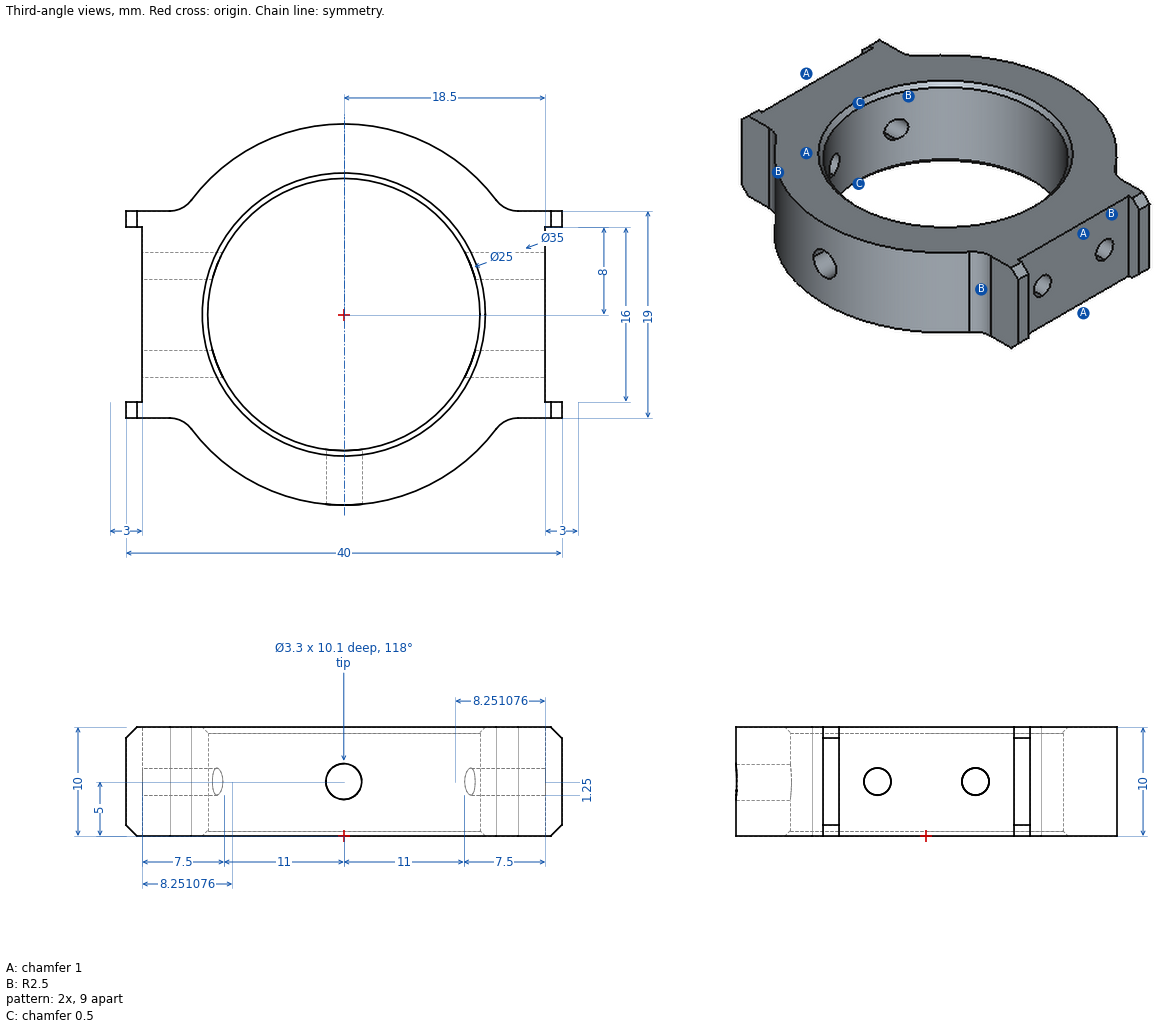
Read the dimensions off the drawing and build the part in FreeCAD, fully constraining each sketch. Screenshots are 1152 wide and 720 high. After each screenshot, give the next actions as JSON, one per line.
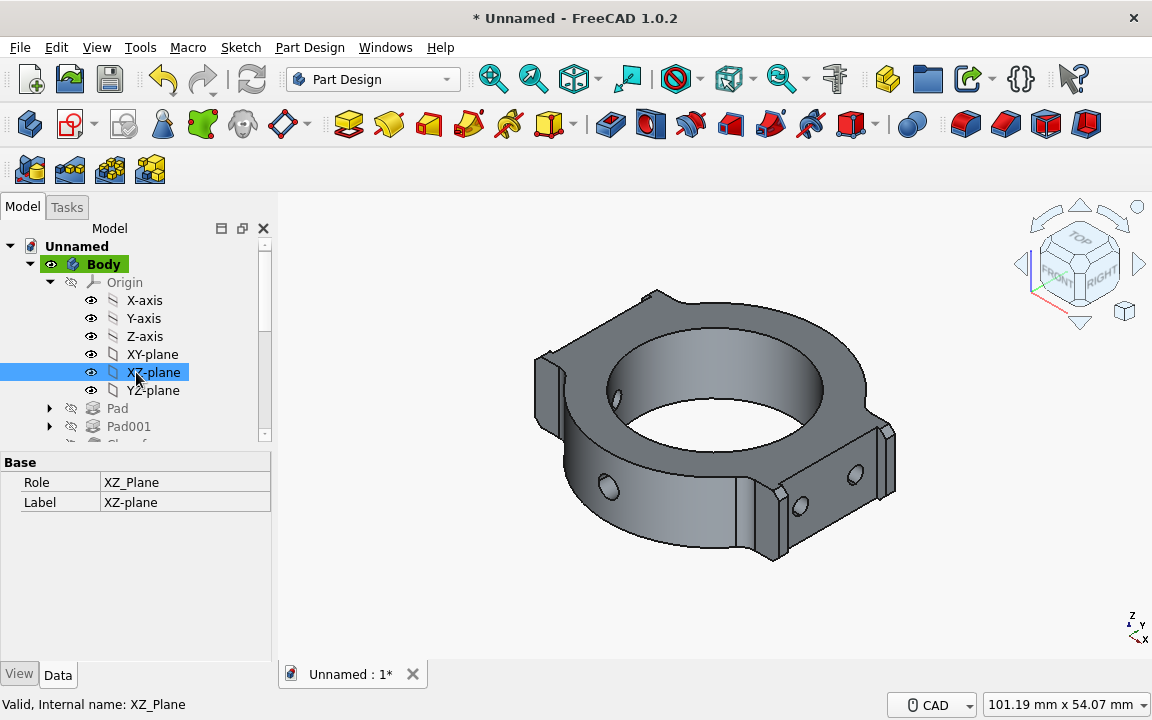
{"action": "left_click", "coordinate": [284, 124]}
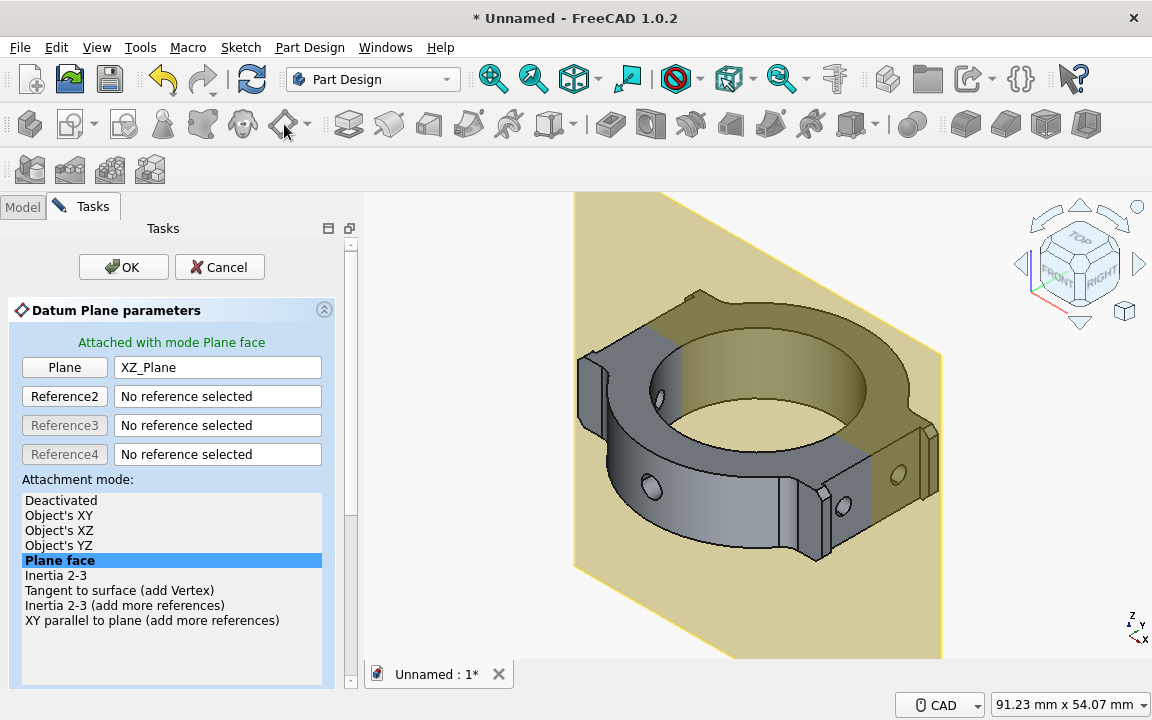
{"action": "scroll", "coordinate": [351, 463], "scroll_direction": "down", "scroll_amount": 3}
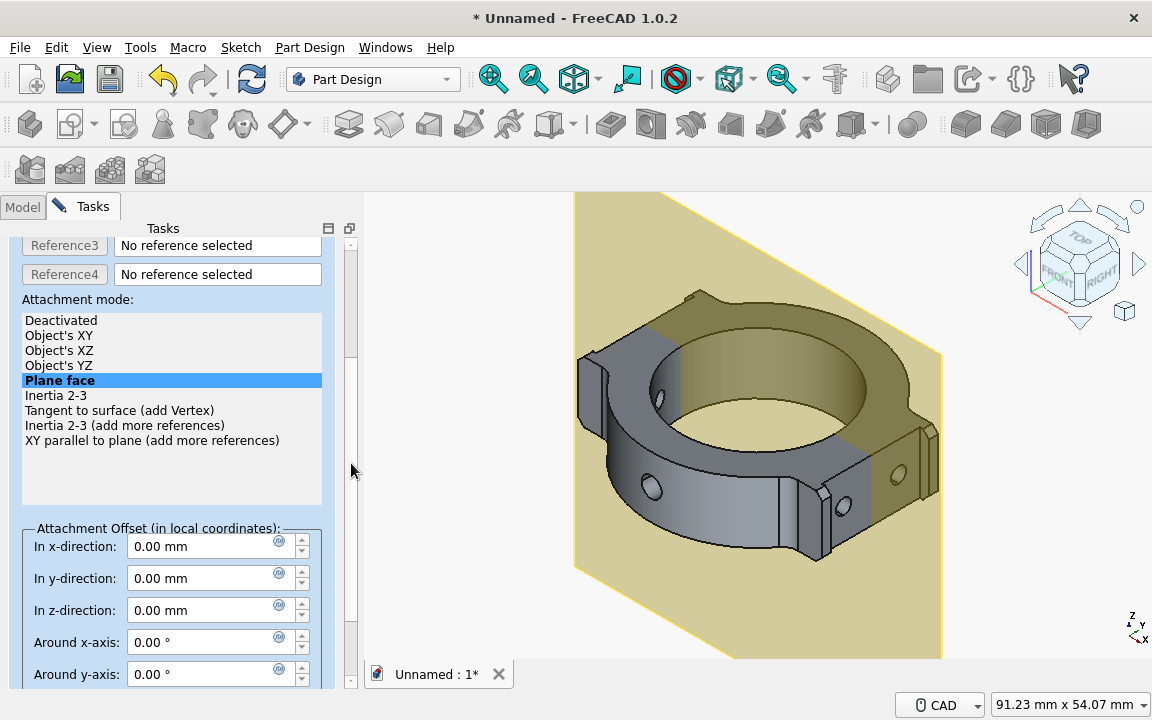
{"action": "triple_click", "coordinate": [210, 610]}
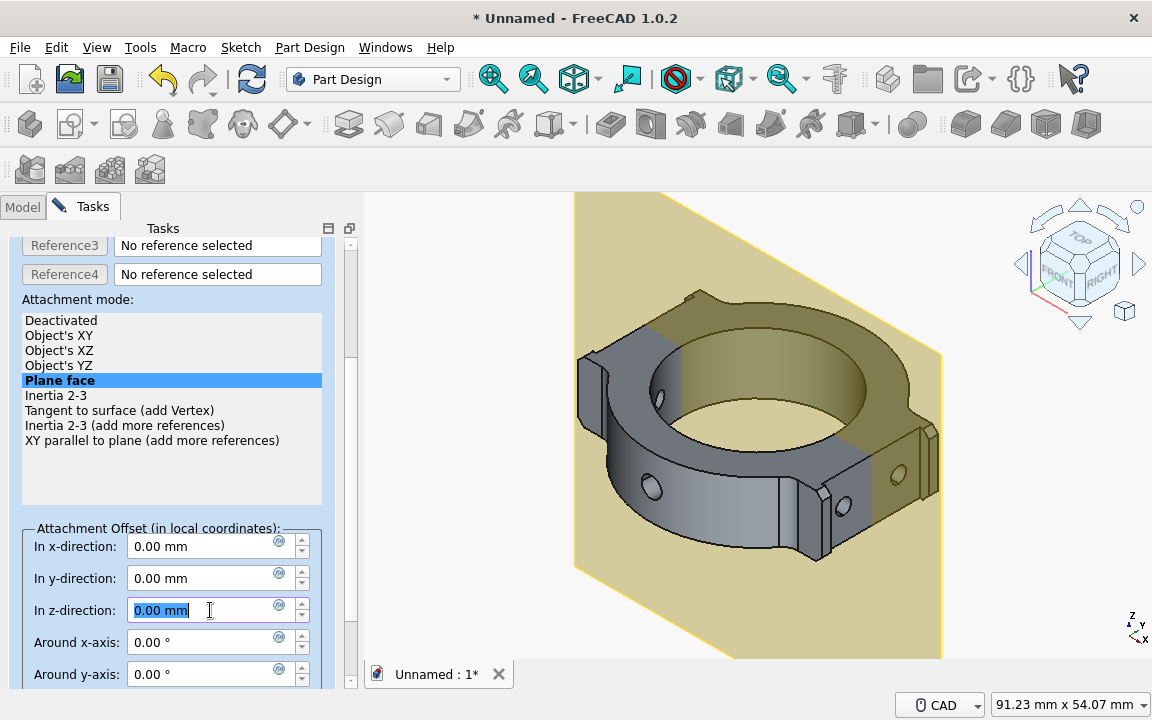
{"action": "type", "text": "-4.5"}
{"action": "key", "text": "Tab"}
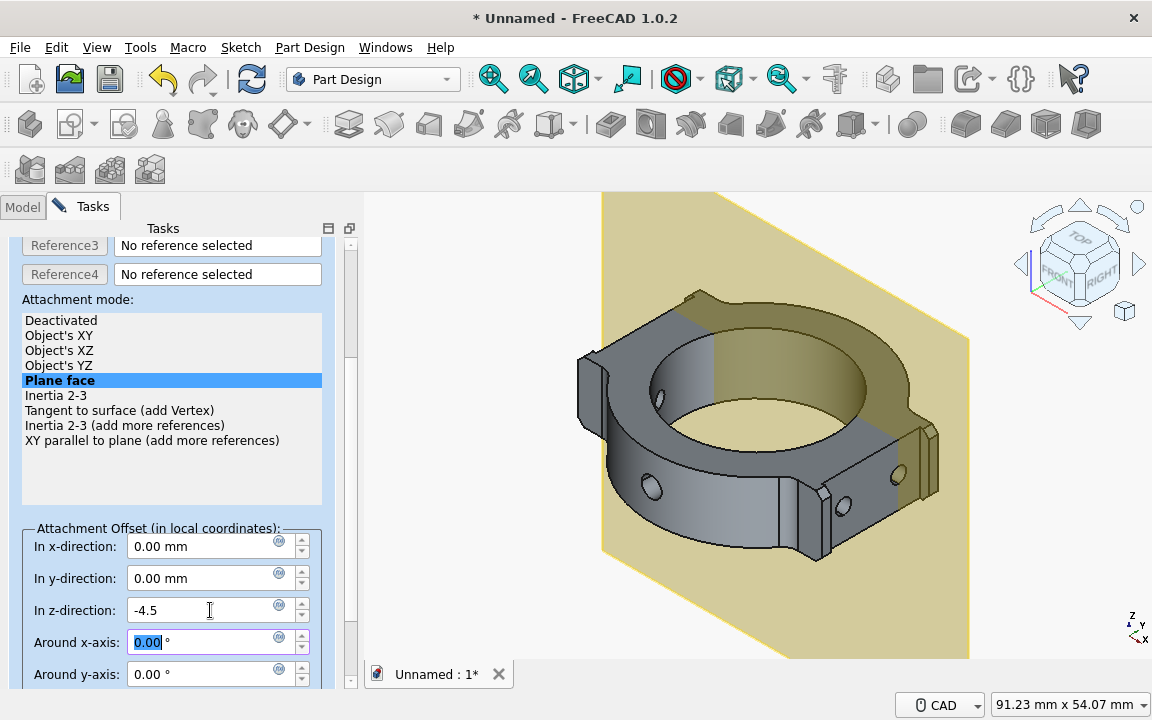
{"action": "scroll", "coordinate": [351, 463], "scroll_direction": "up", "scroll_amount": 4}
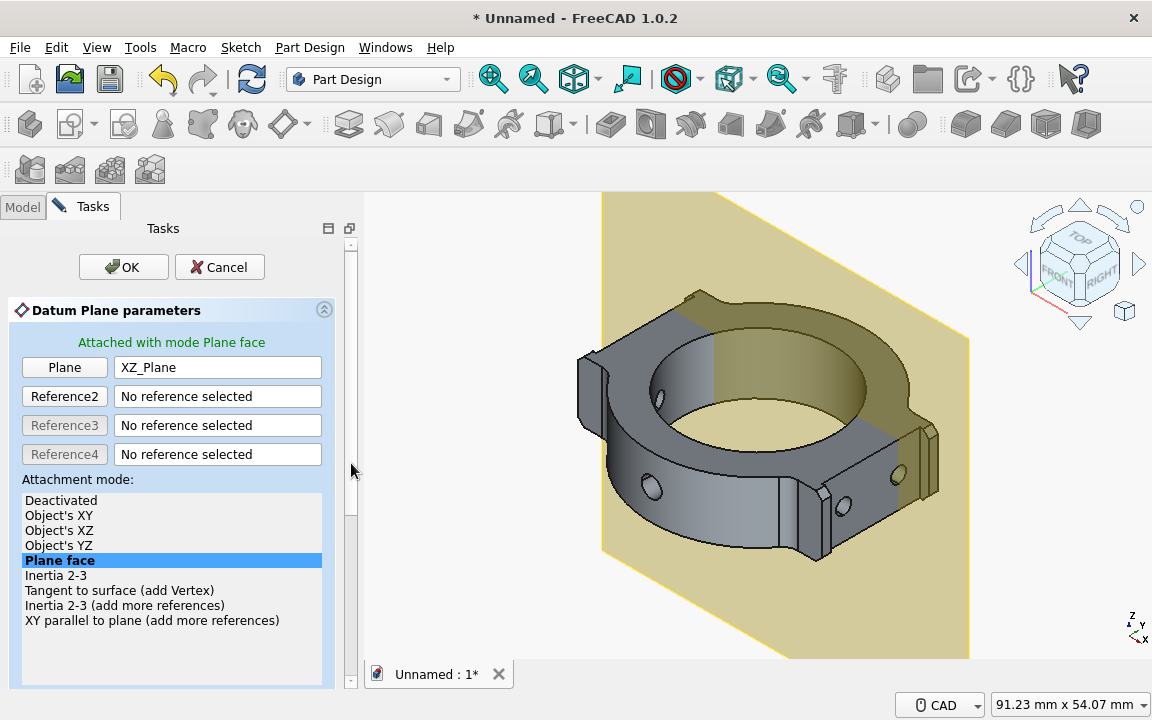
{"action": "left_click", "coordinate": [124, 267]}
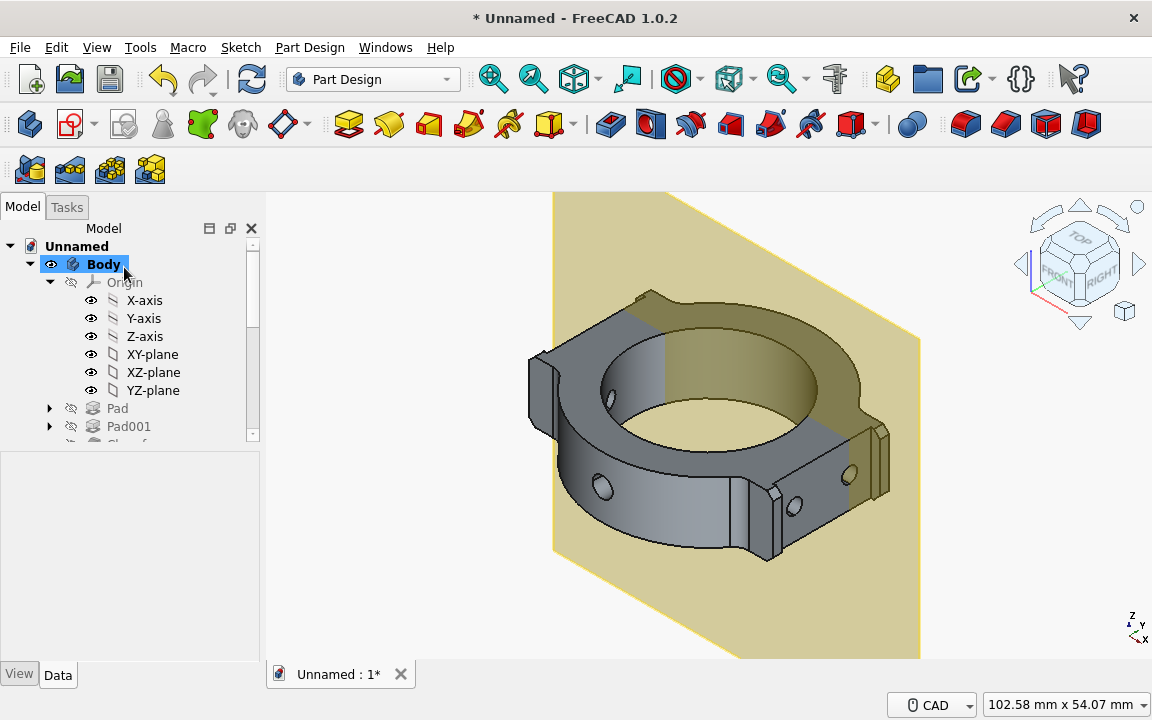
{"action": "scroll", "coordinate": [100, 332], "scroll_direction": "down", "scroll_amount": 3}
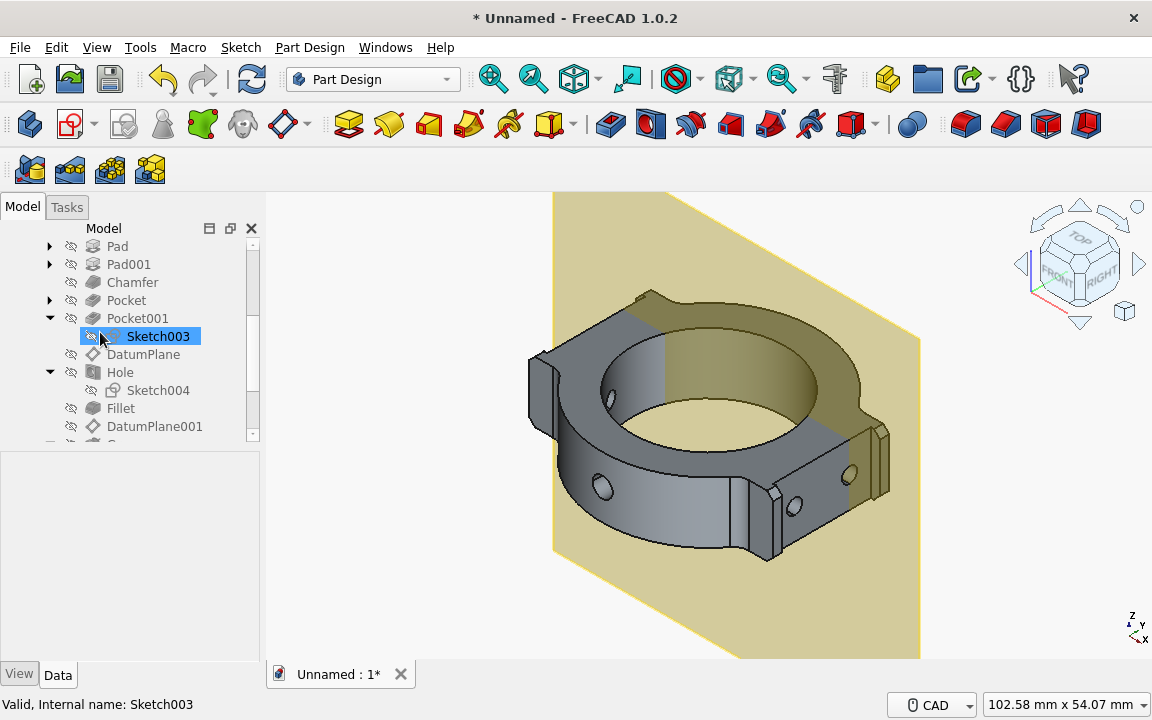
{"action": "scroll", "coordinate": [140, 332], "scroll_direction": "up", "scroll_amount": 15}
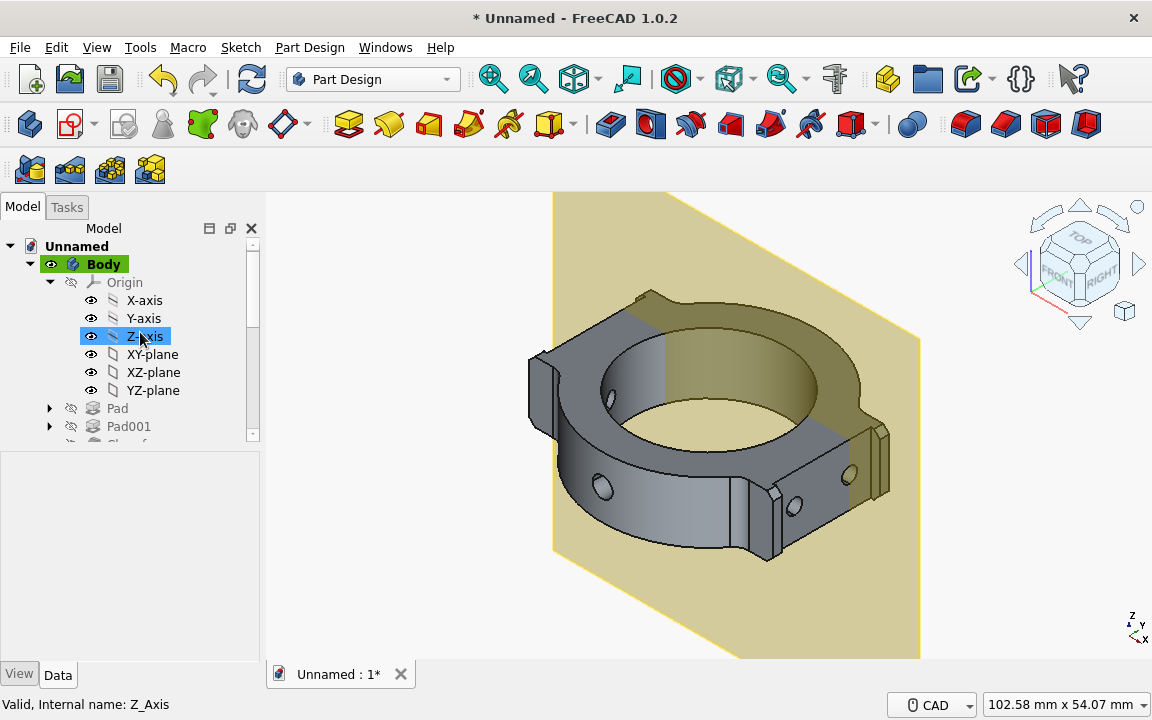
{"action": "scroll", "coordinate": [100, 332], "scroll_direction": "down", "scroll_amount": 6}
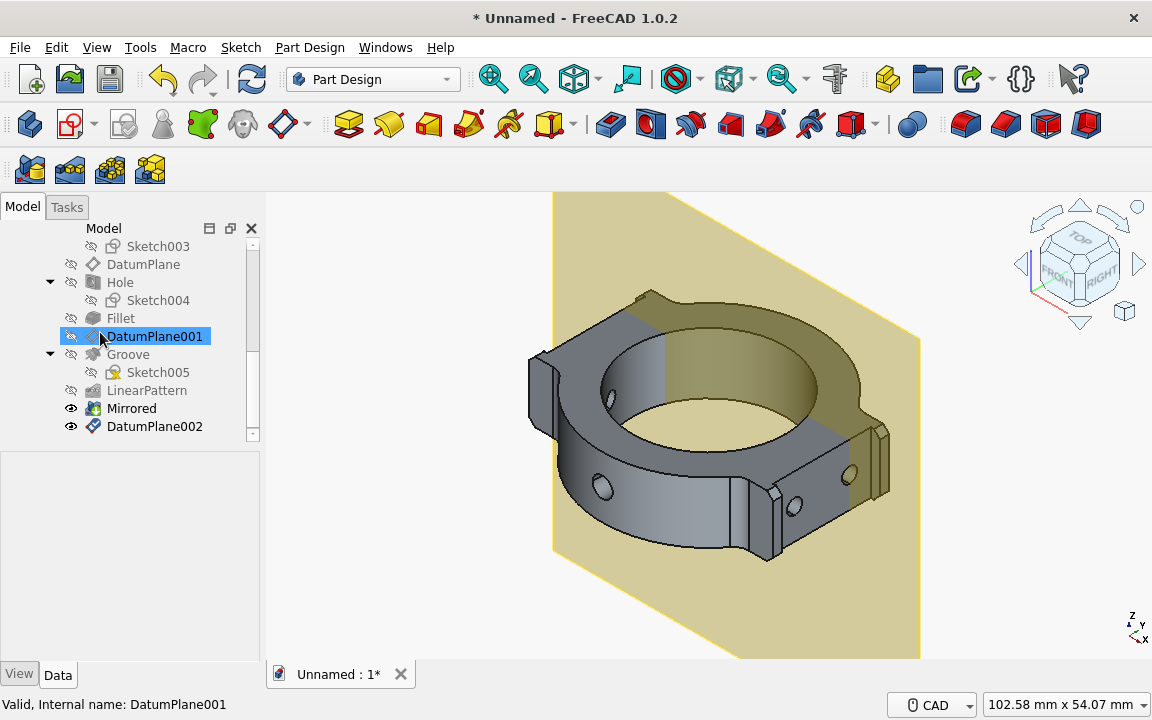
{"action": "left_click", "coordinate": [116, 426]}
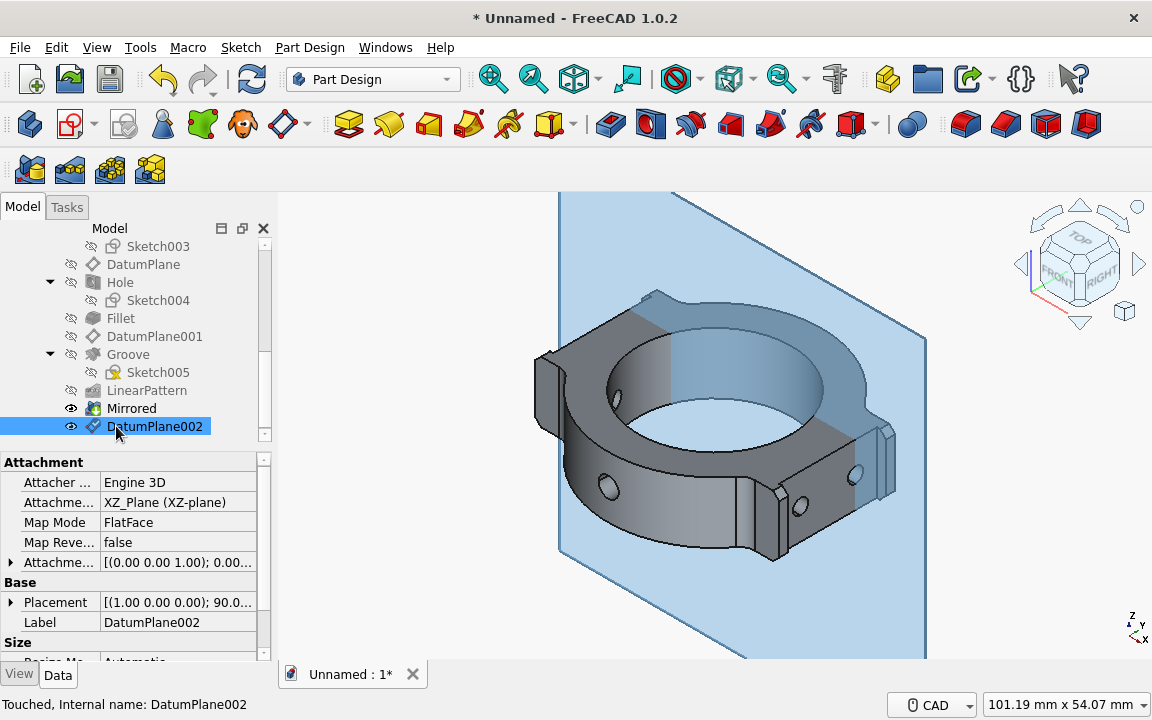
{"action": "left_click", "coordinate": [70, 124]}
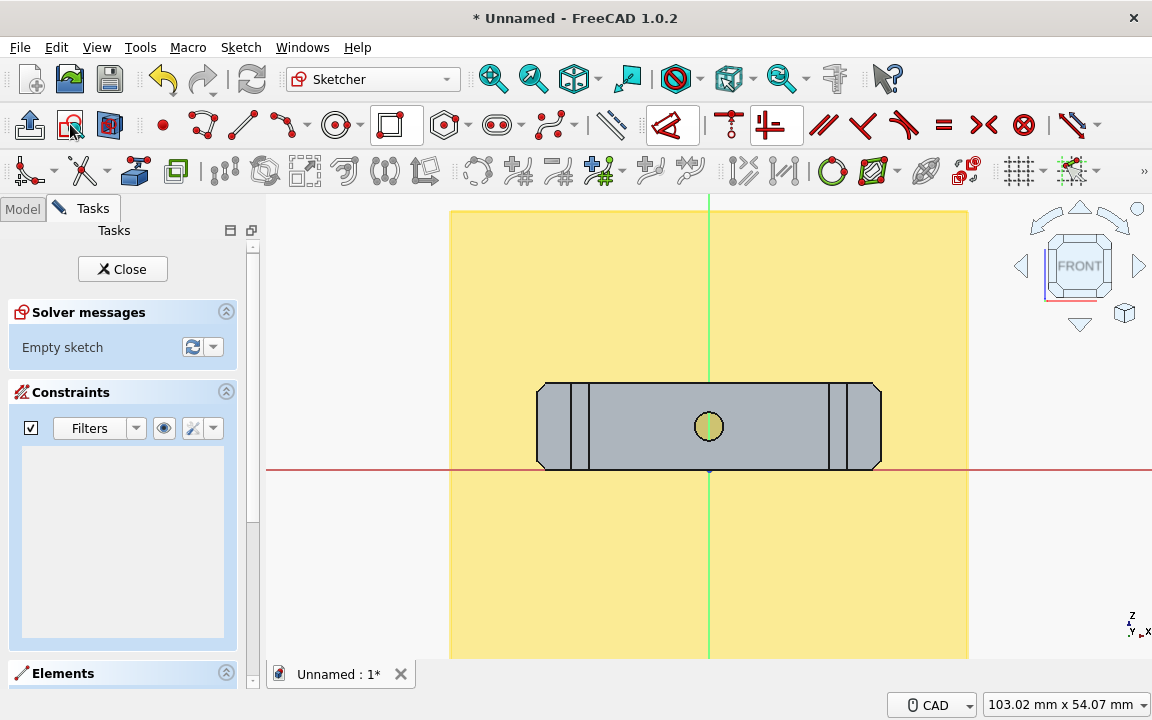
{"action": "key", "text": "q s"}